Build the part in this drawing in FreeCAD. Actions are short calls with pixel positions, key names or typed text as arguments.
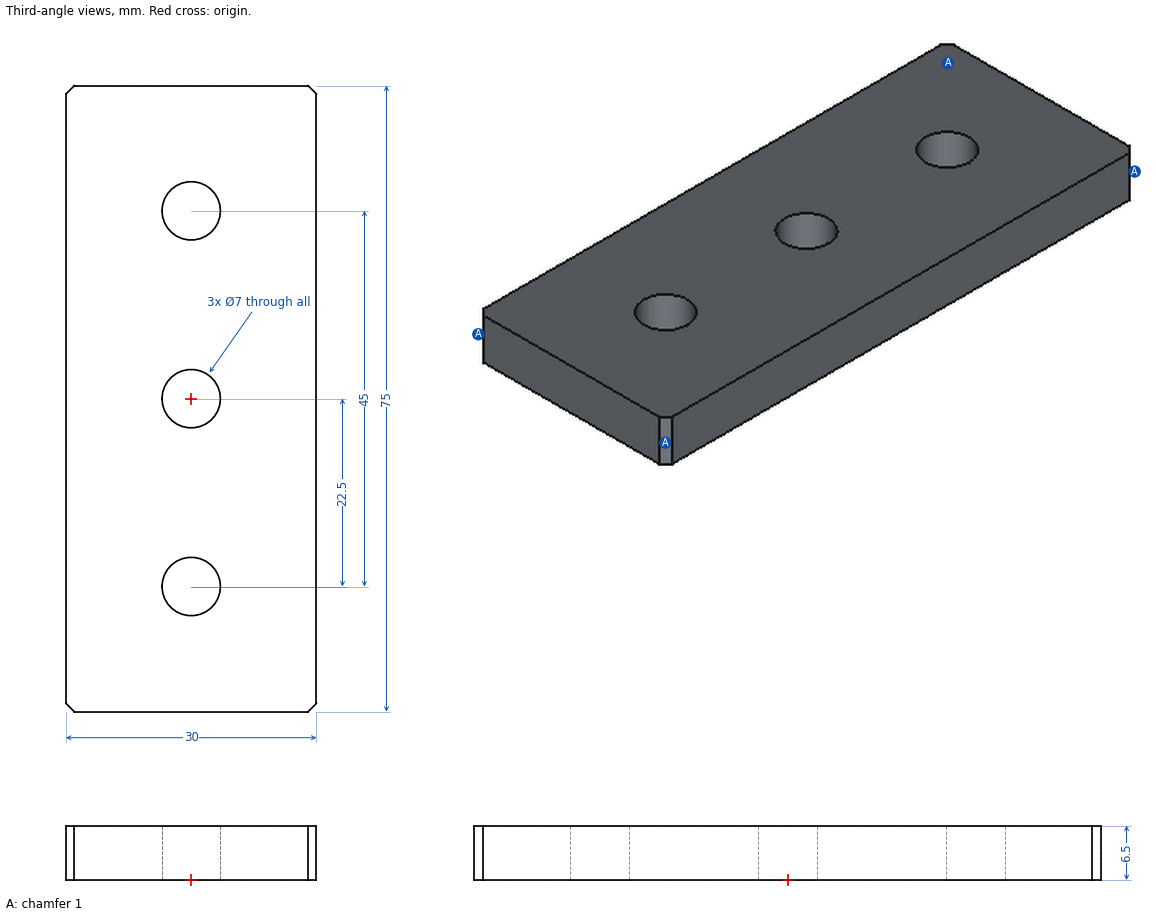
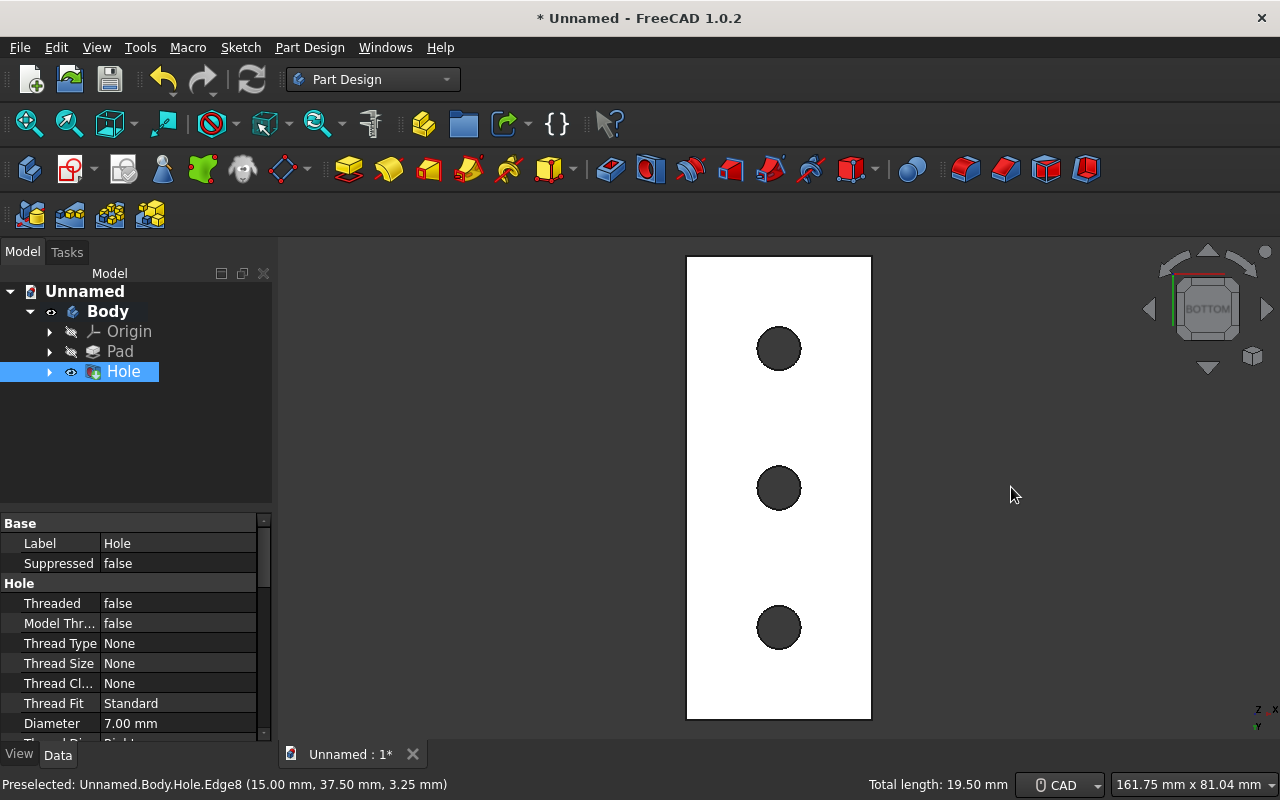
key(4)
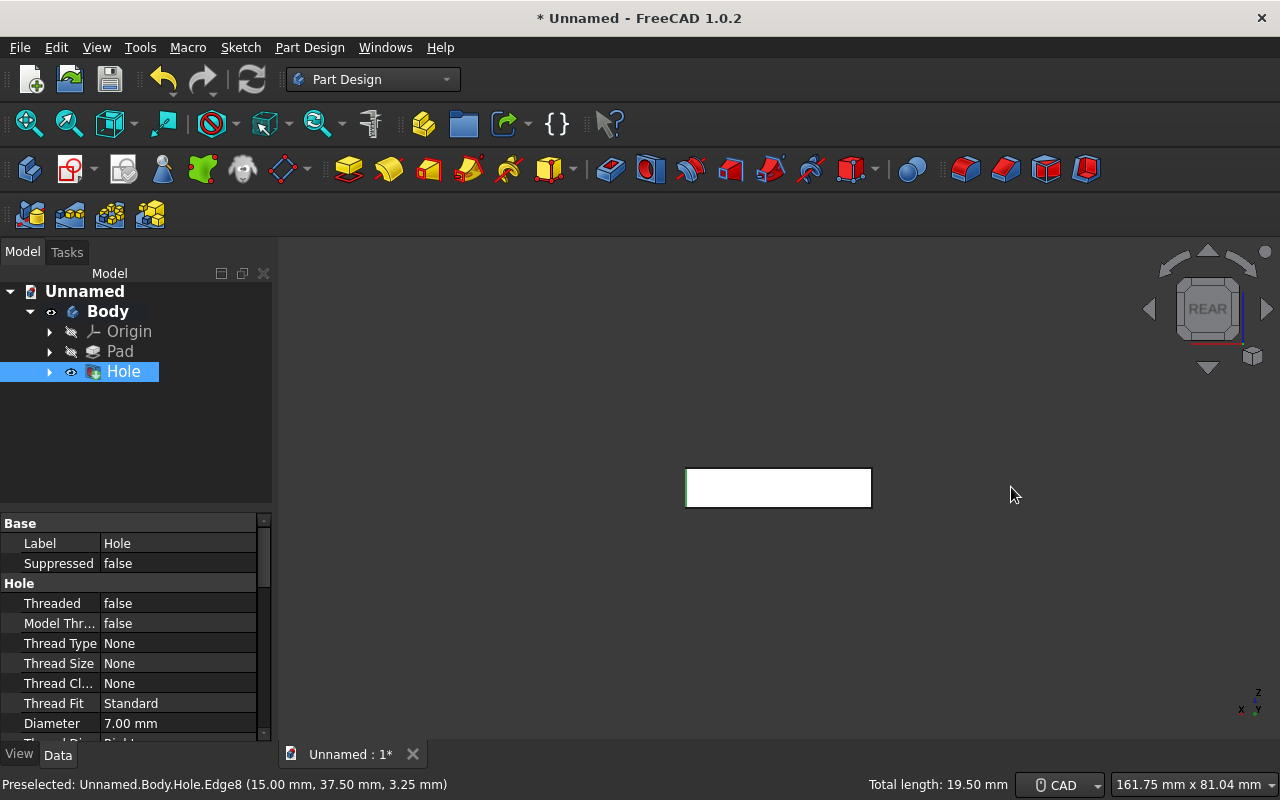
key(v)
key(f)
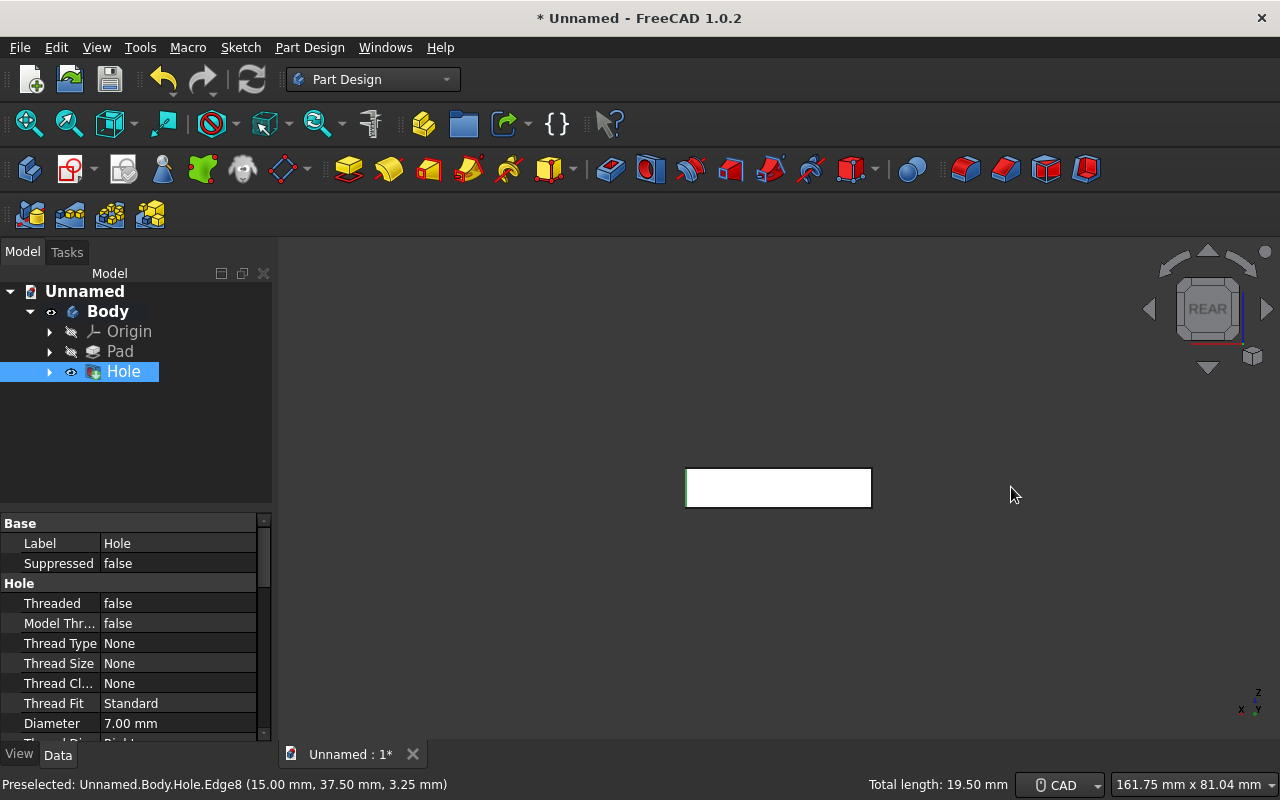
click(872, 487, ctrl)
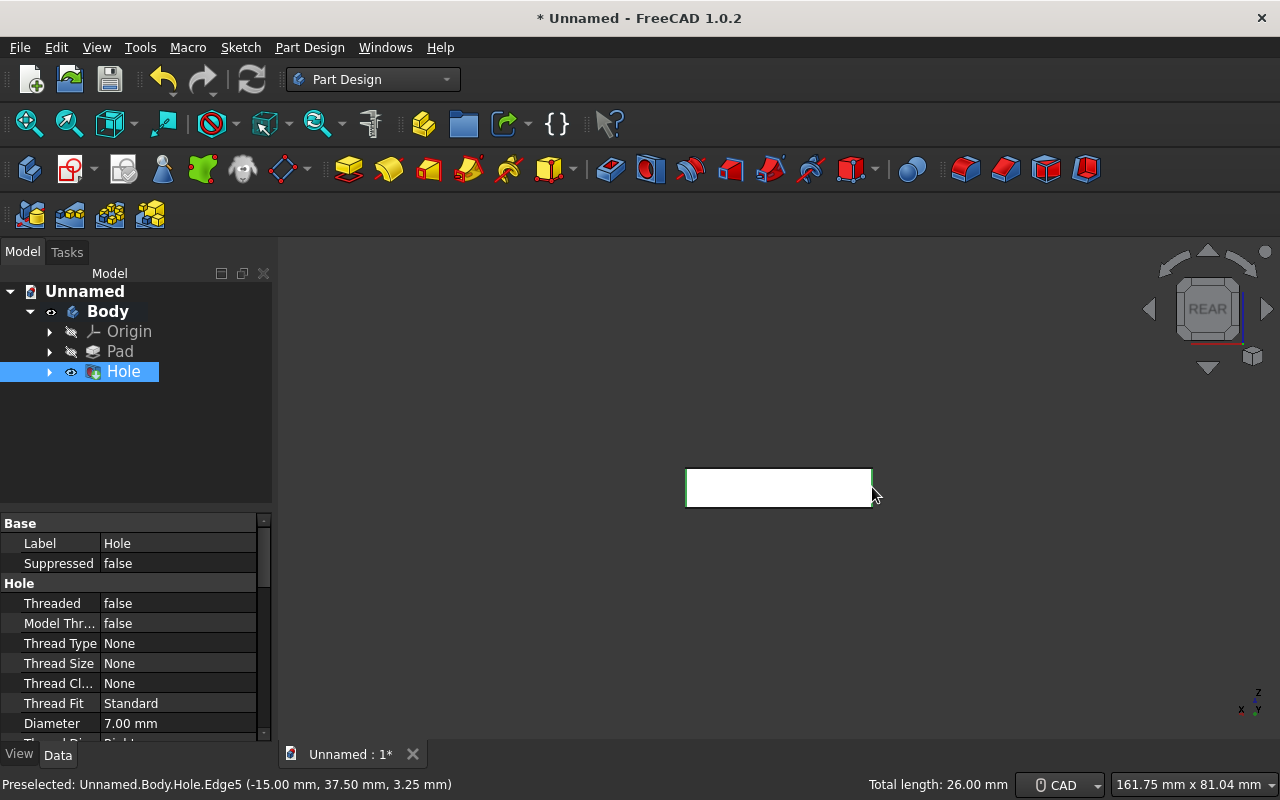
click(1006, 170)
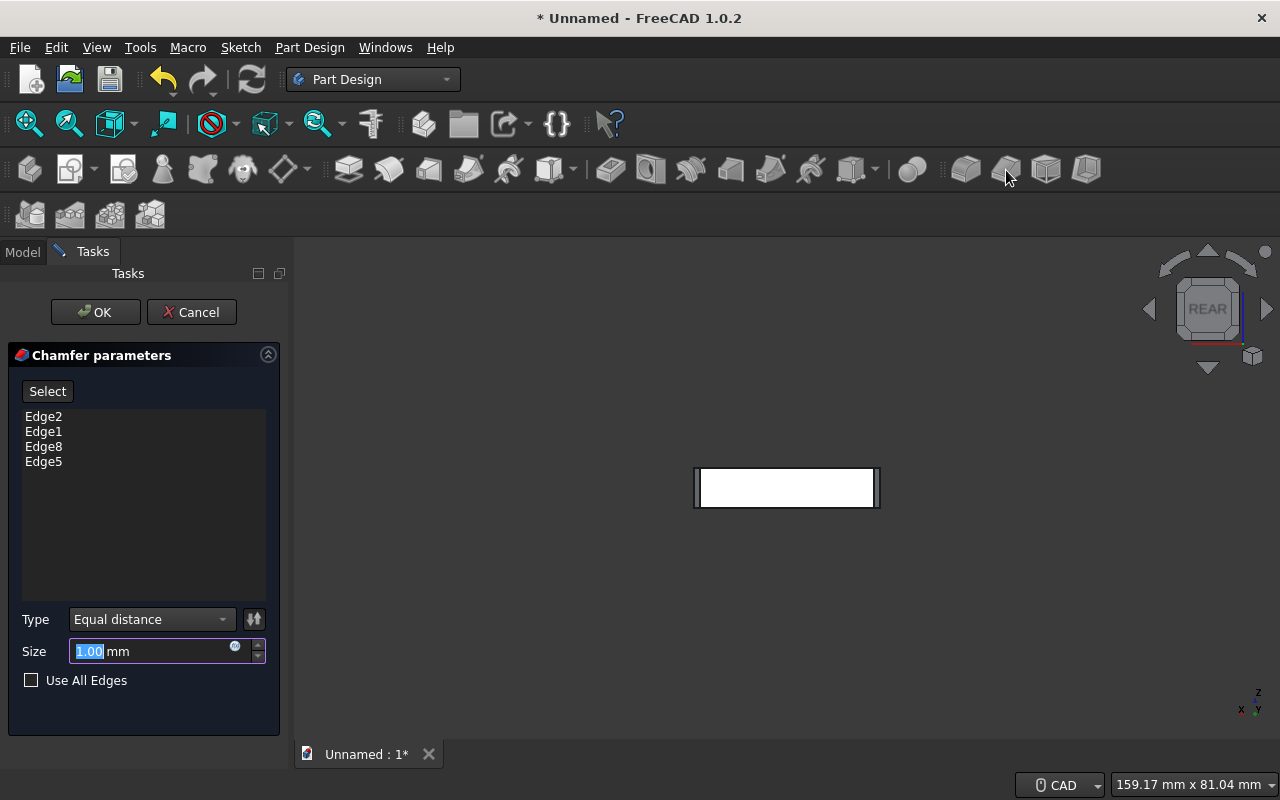
text(1)
key(Tab)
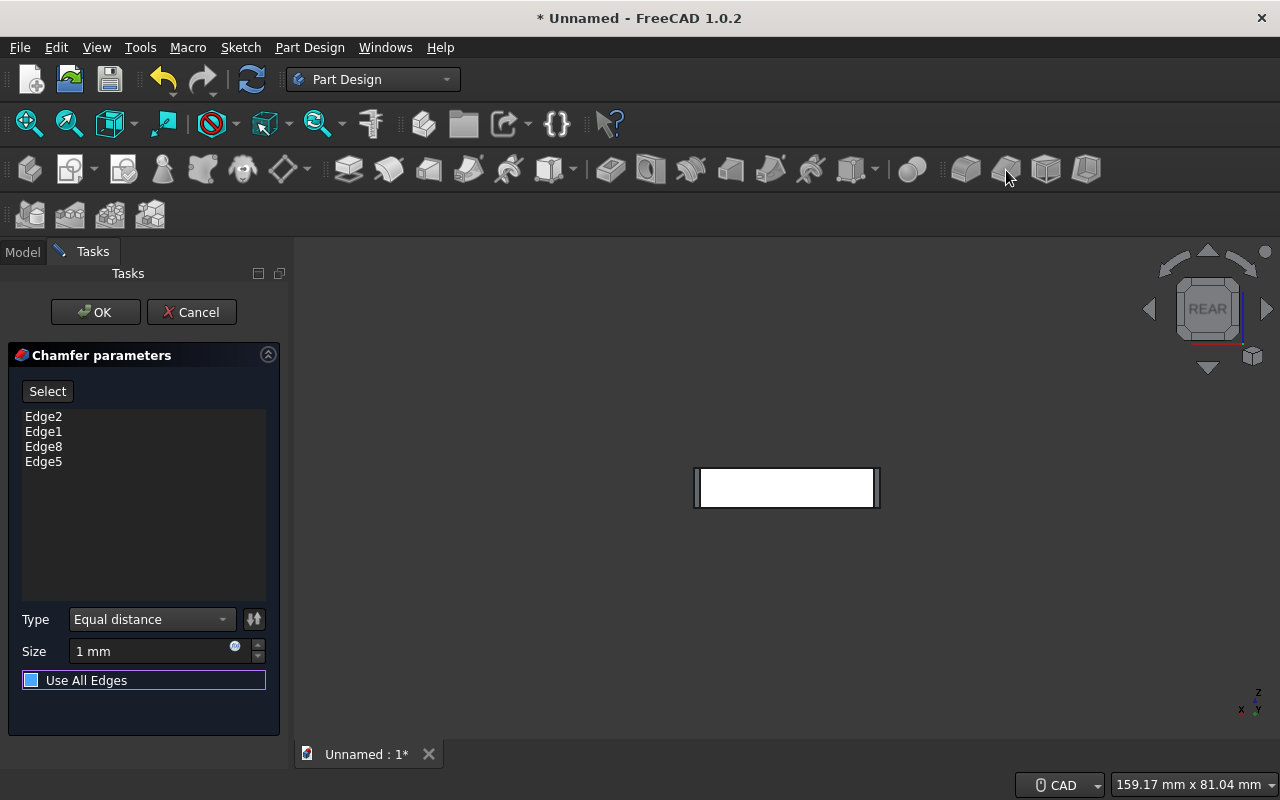
click(96, 312)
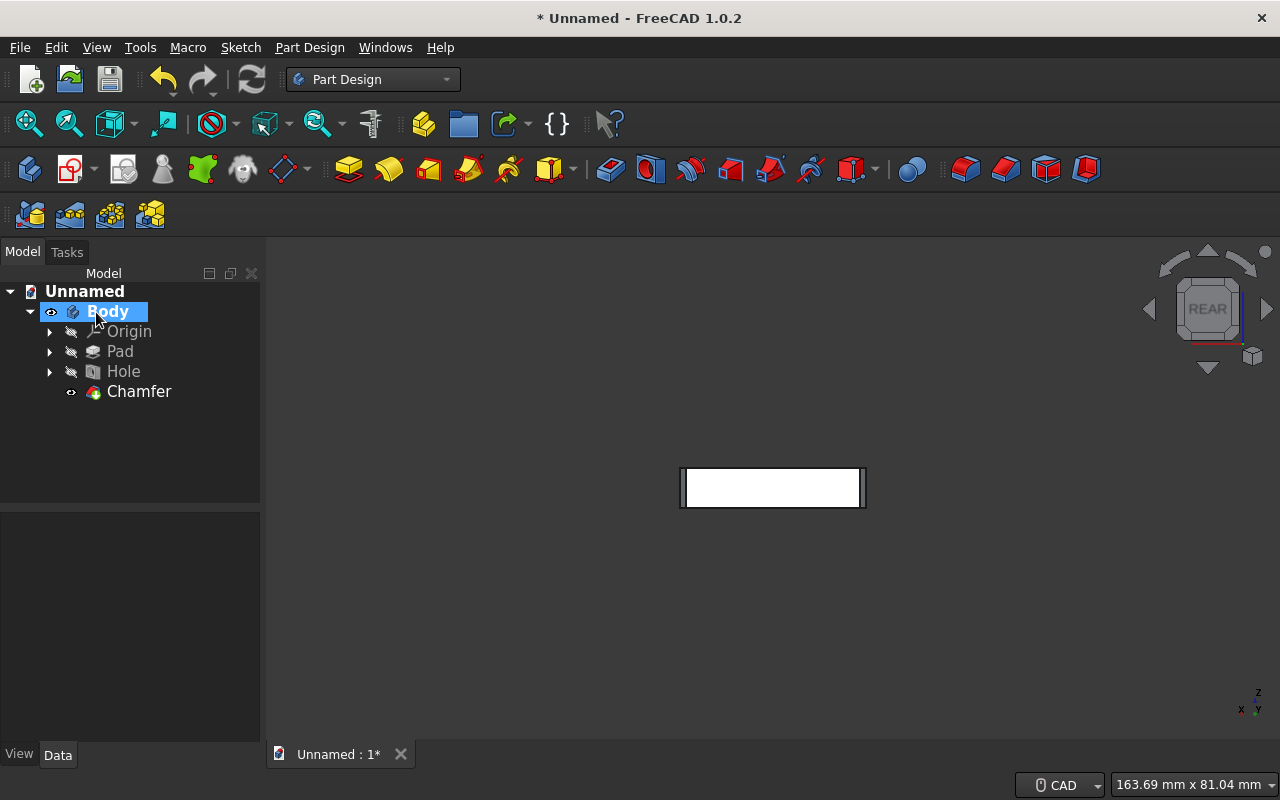
key(0)